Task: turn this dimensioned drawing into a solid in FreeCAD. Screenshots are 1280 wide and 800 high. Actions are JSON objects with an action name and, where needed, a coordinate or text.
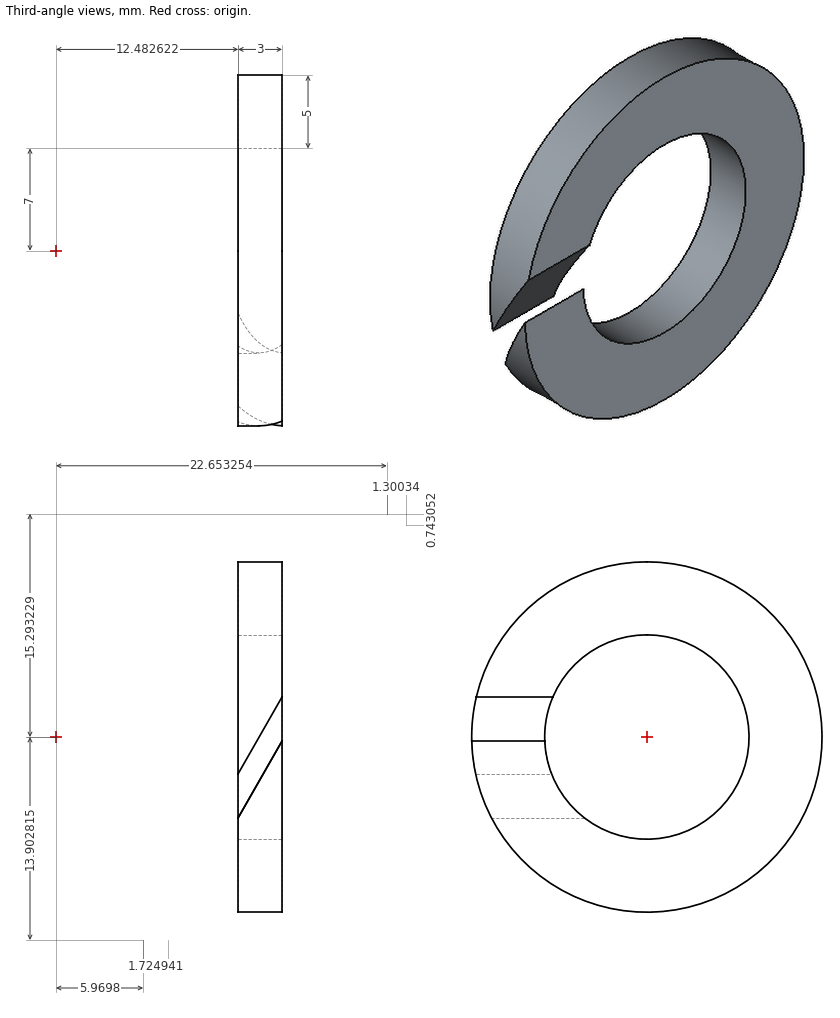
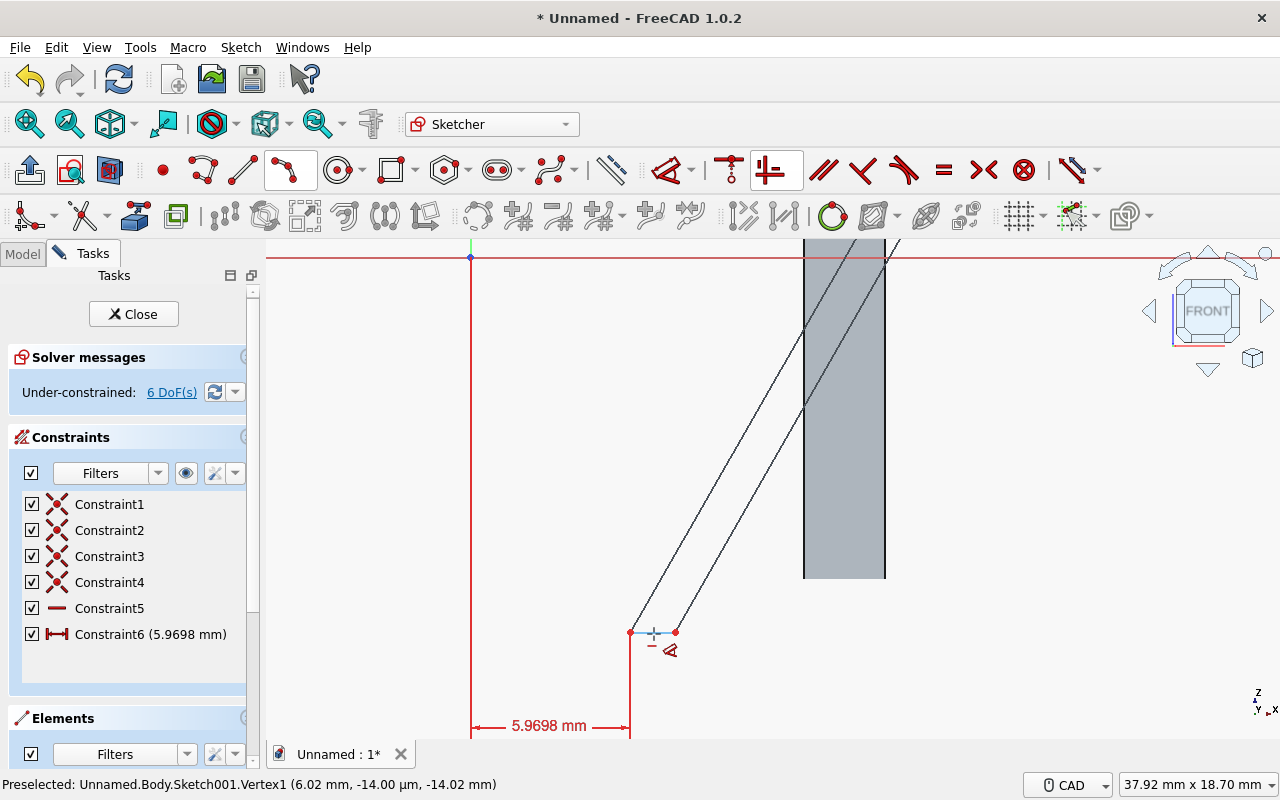
{"action": "left_click", "coordinate": [653, 633]}
{"action": "left_click", "coordinate": [653, 667]}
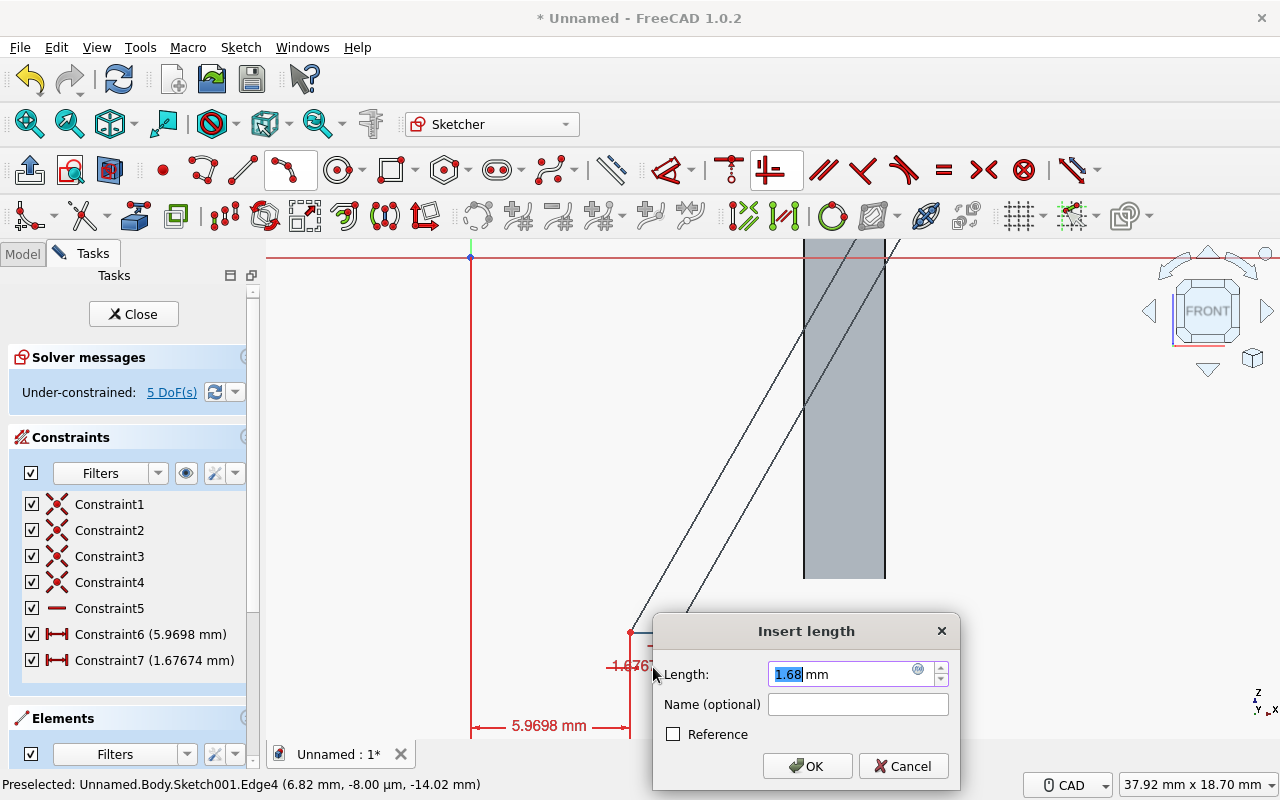
{"action": "type", "text": "1.724941"}
{"action": "key", "text": "Return"}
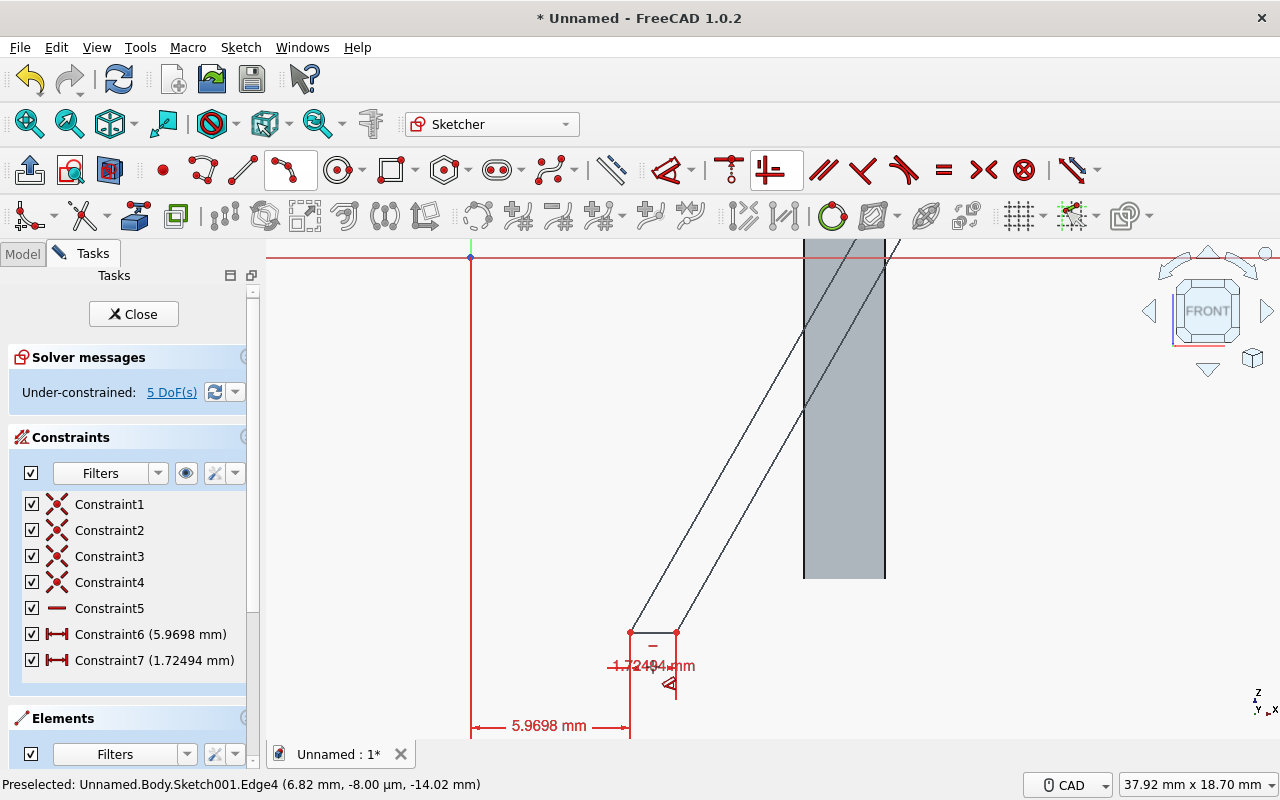
{"action": "scroll", "coordinate": [654, 634], "scroll_direction": "down", "scroll_amount": 5}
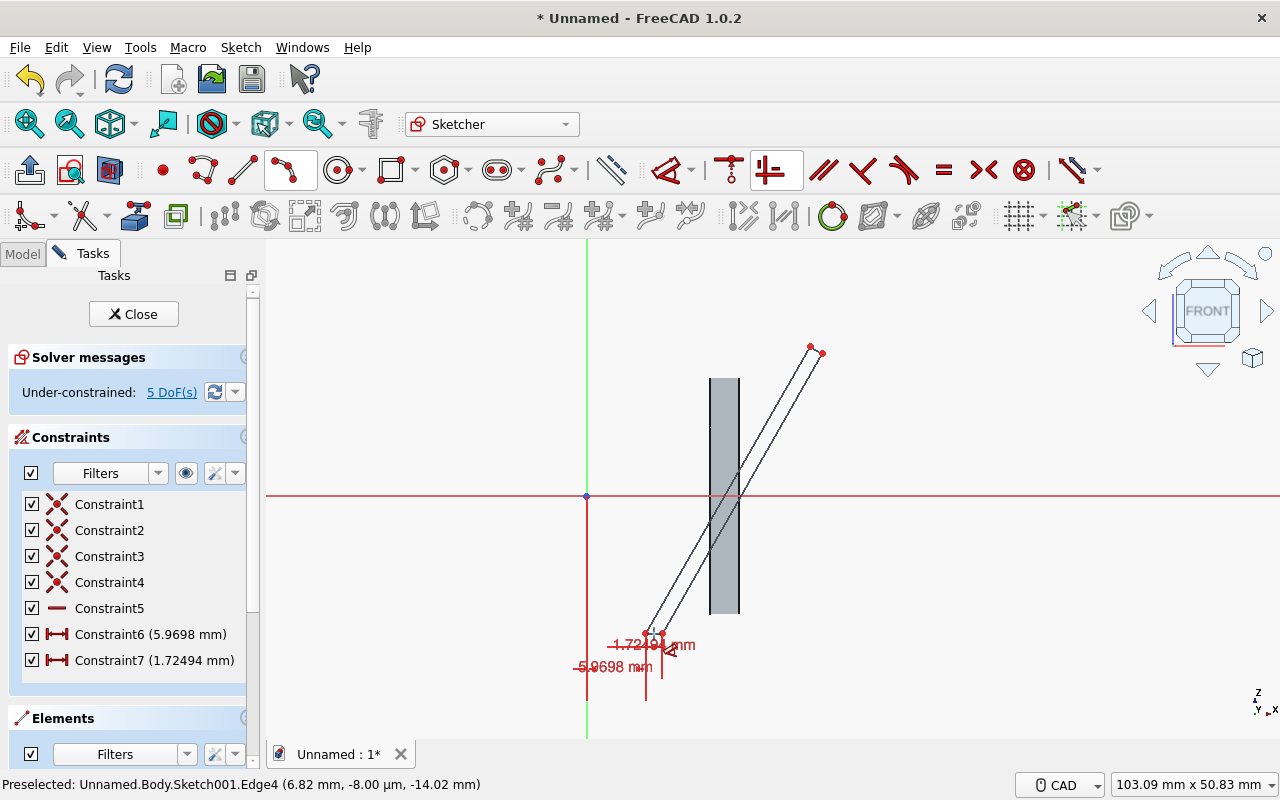
{"action": "scroll", "coordinate": [814, 349], "scroll_direction": "up", "scroll_amount": 6}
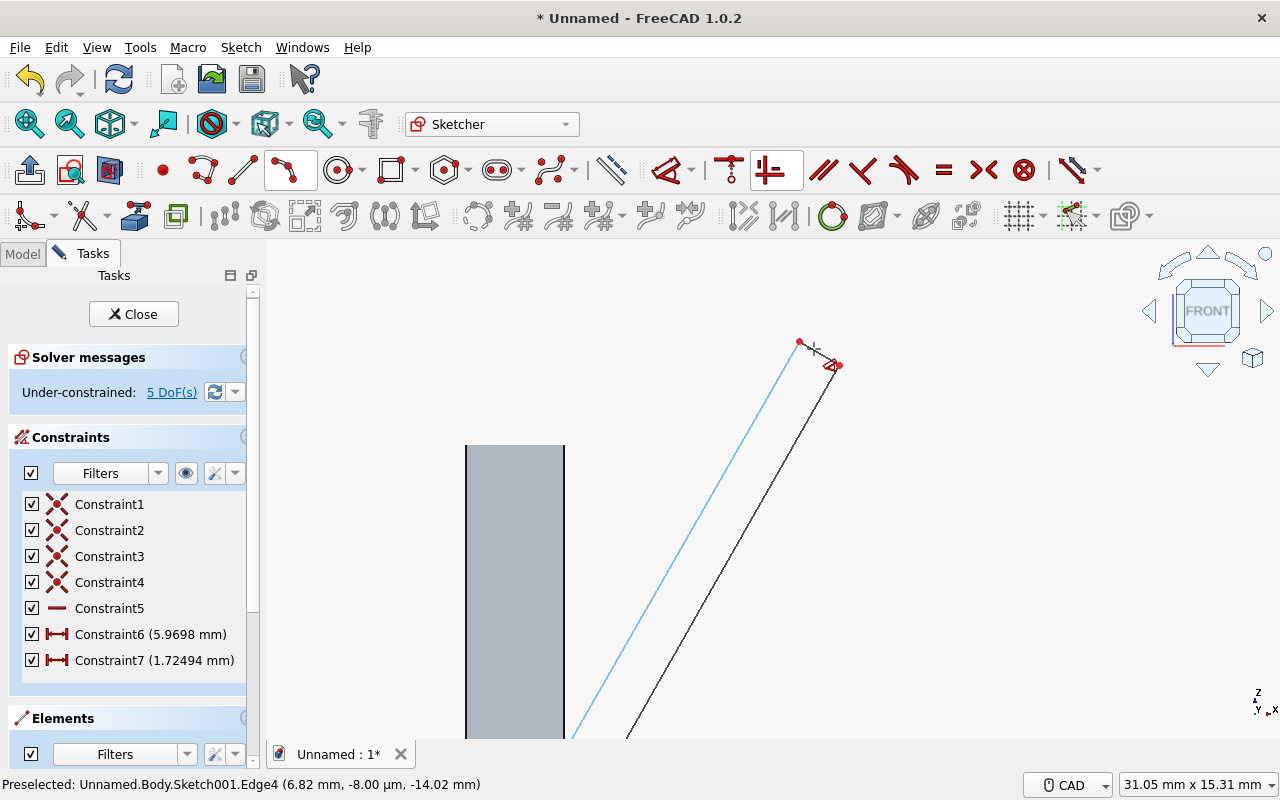
{"action": "left_click", "coordinate": [811, 349]}
{"action": "left_click", "coordinate": [819, 308]}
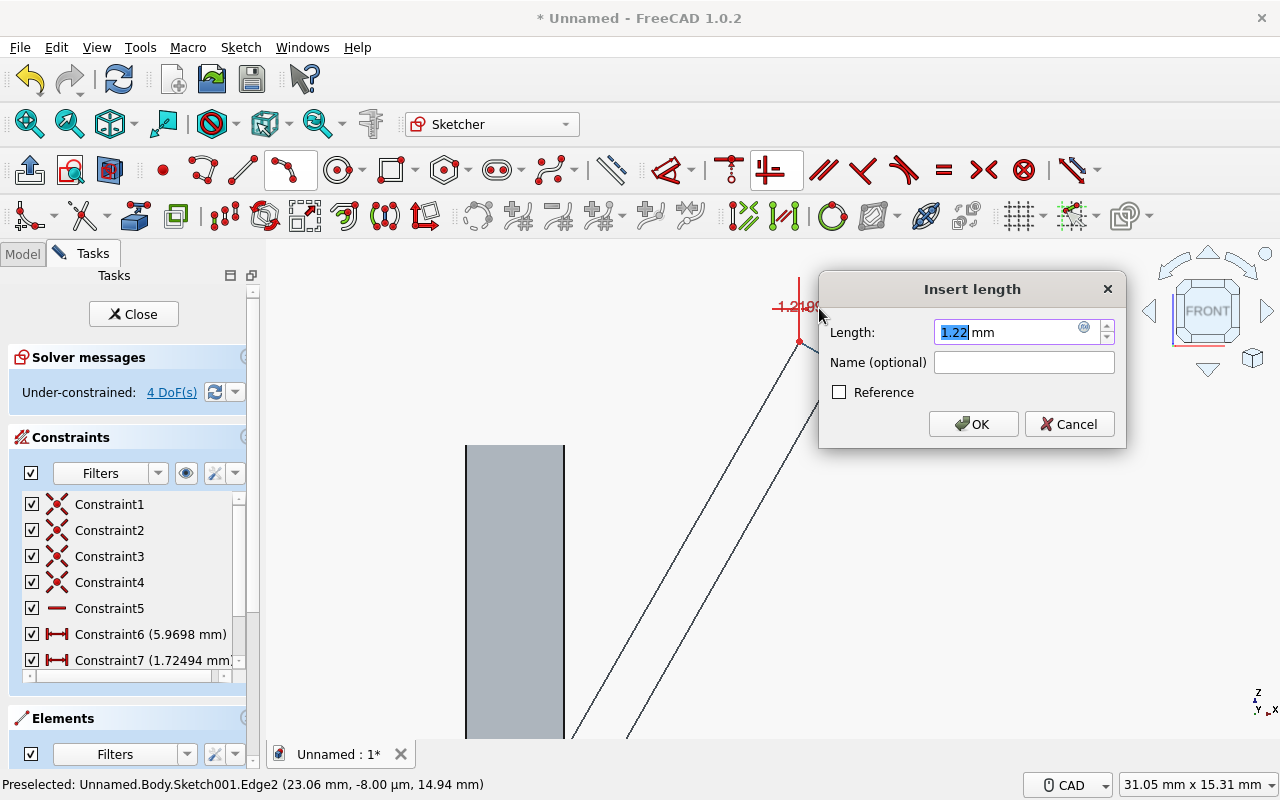
{"action": "type", "text": "1.30034"}
{"action": "key", "text": "Return"}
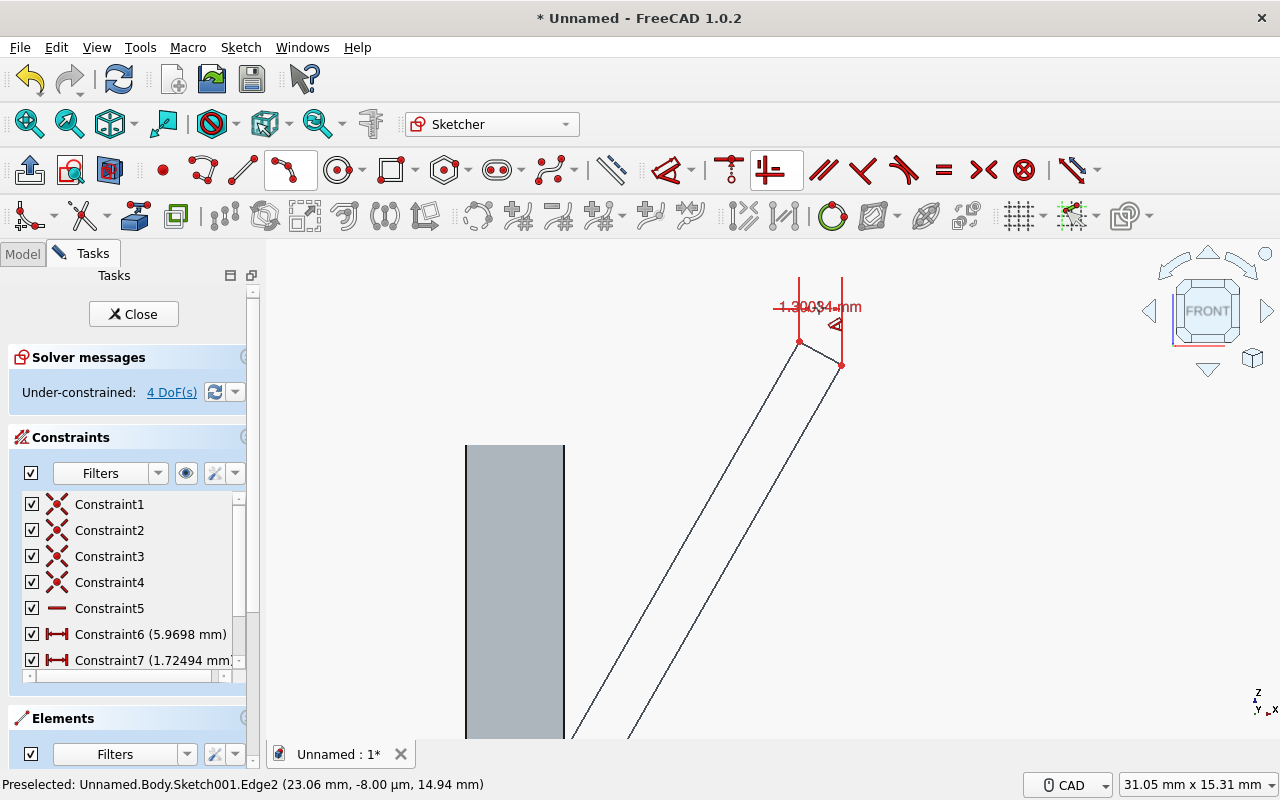
{"action": "scroll", "coordinate": [812, 349], "scroll_direction": "up", "scroll_amount": 3}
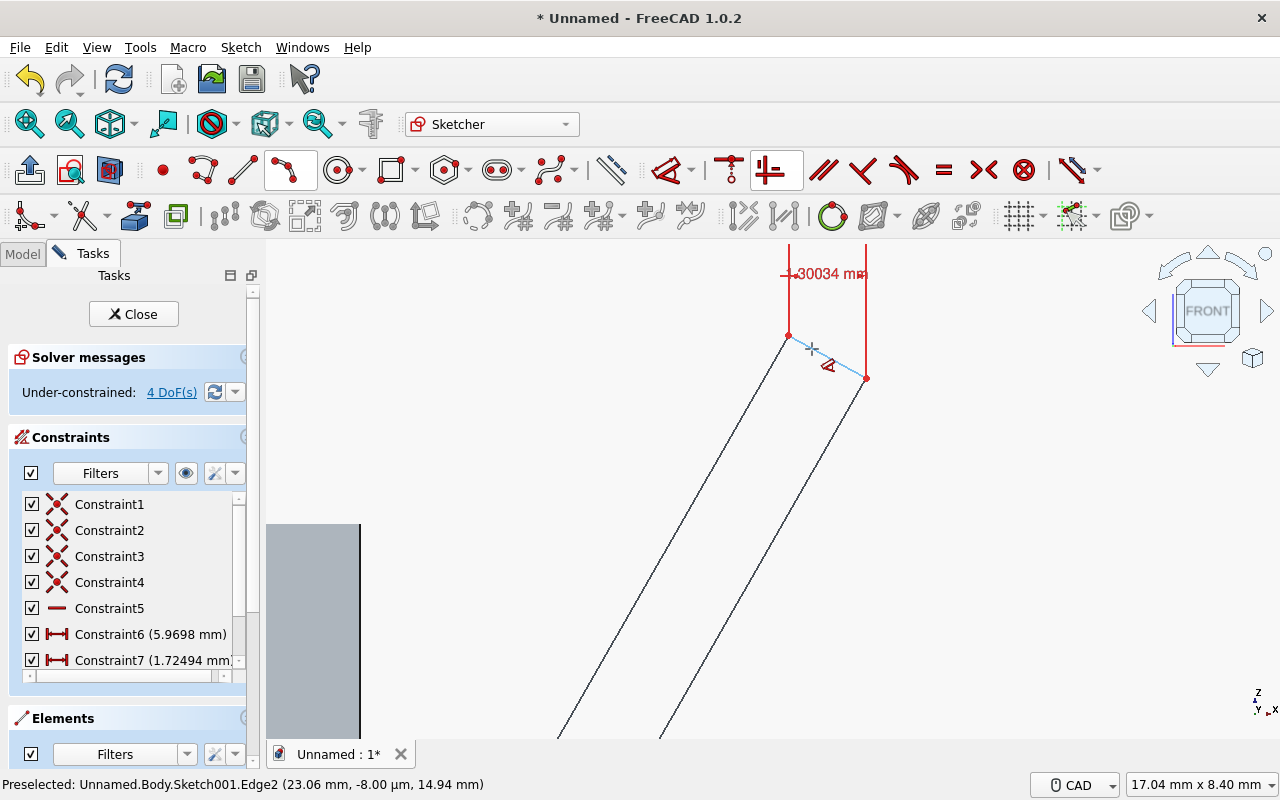
{"action": "left_click", "coordinate": [812, 348]}
{"action": "left_click", "coordinate": [900, 357]}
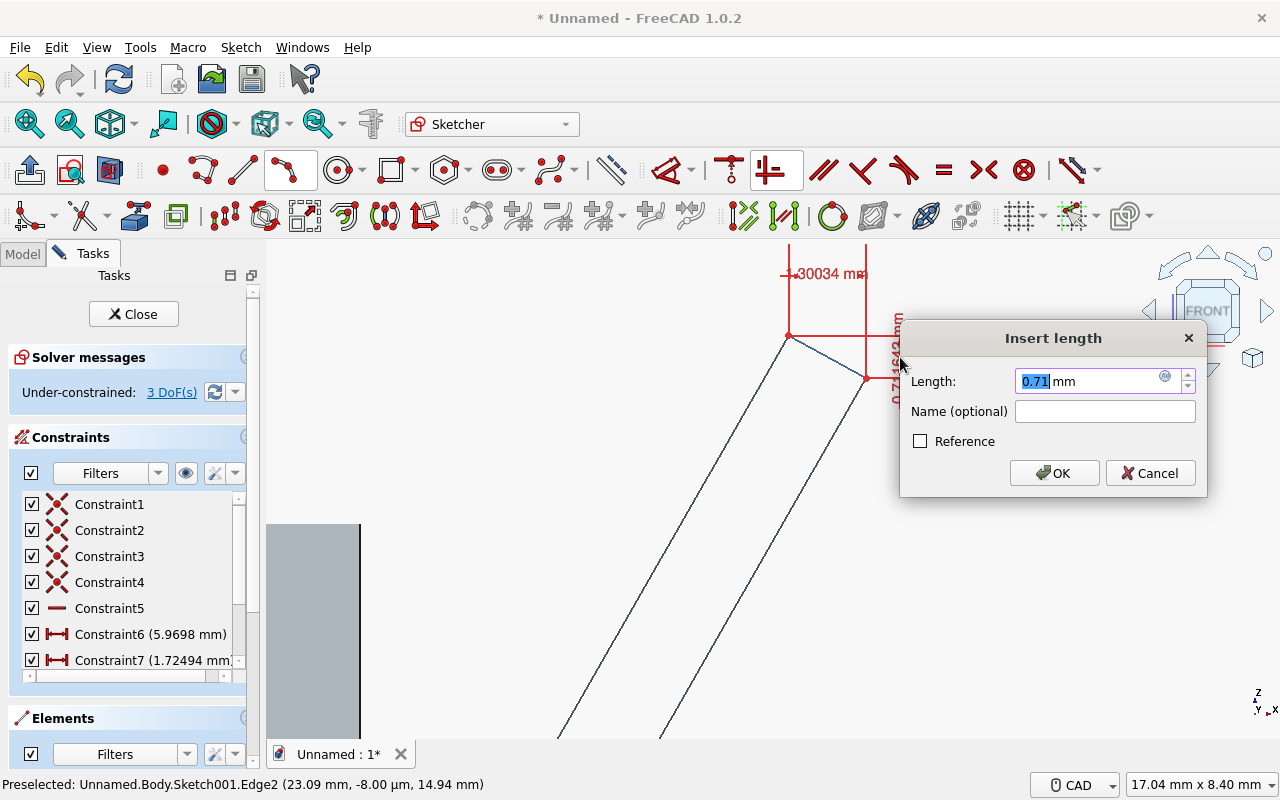
{"action": "type", "text": "0.743052"}
{"action": "key", "text": "Return"}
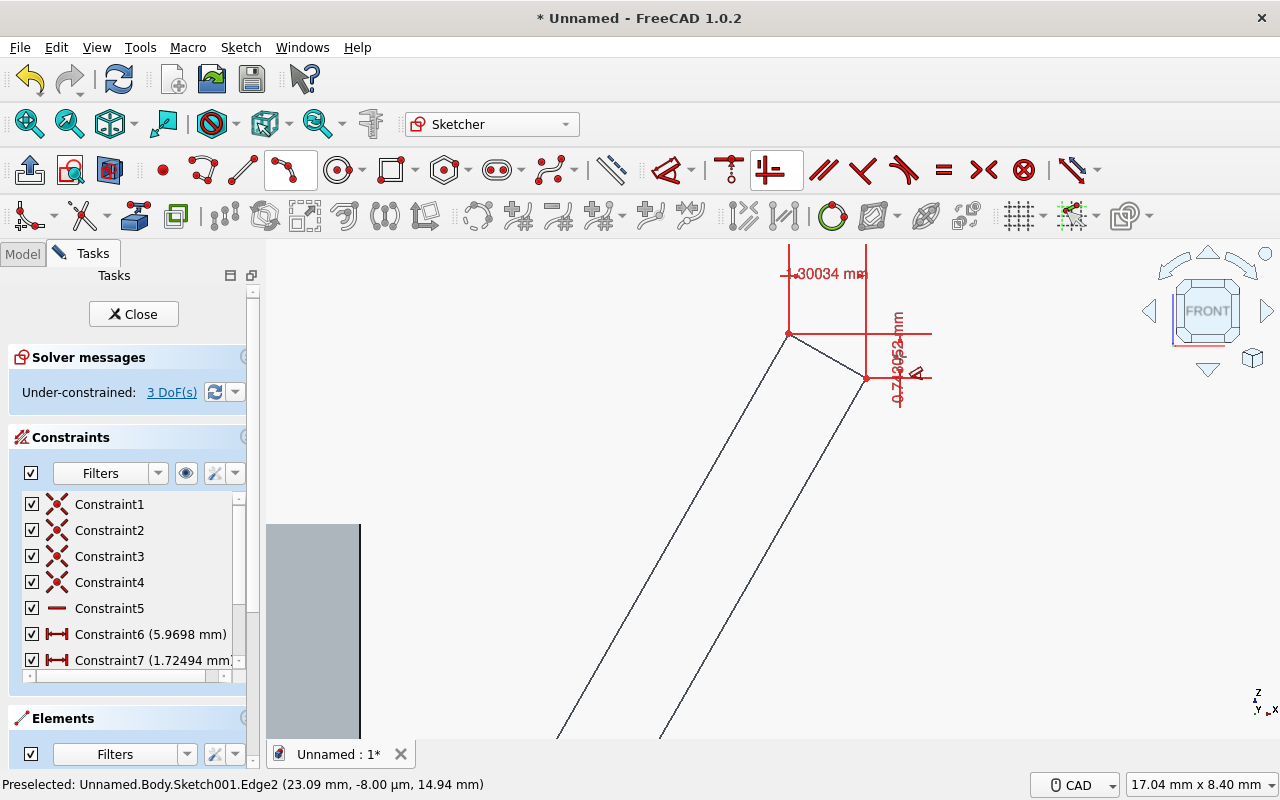
{"action": "scroll", "coordinate": [814, 349], "scroll_direction": "down", "scroll_amount": 9}